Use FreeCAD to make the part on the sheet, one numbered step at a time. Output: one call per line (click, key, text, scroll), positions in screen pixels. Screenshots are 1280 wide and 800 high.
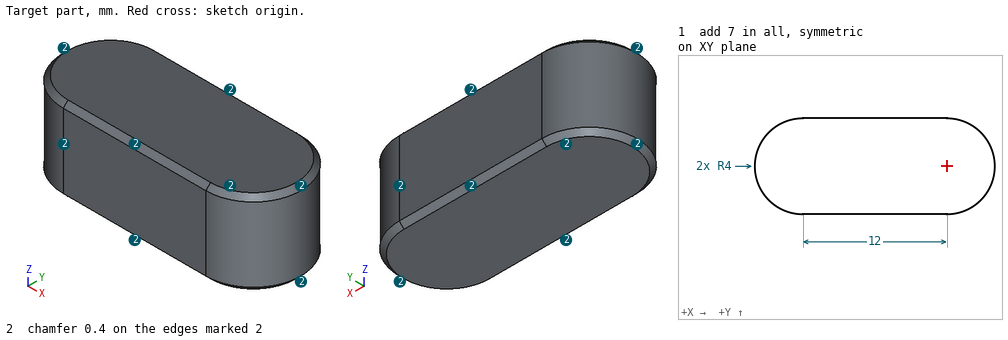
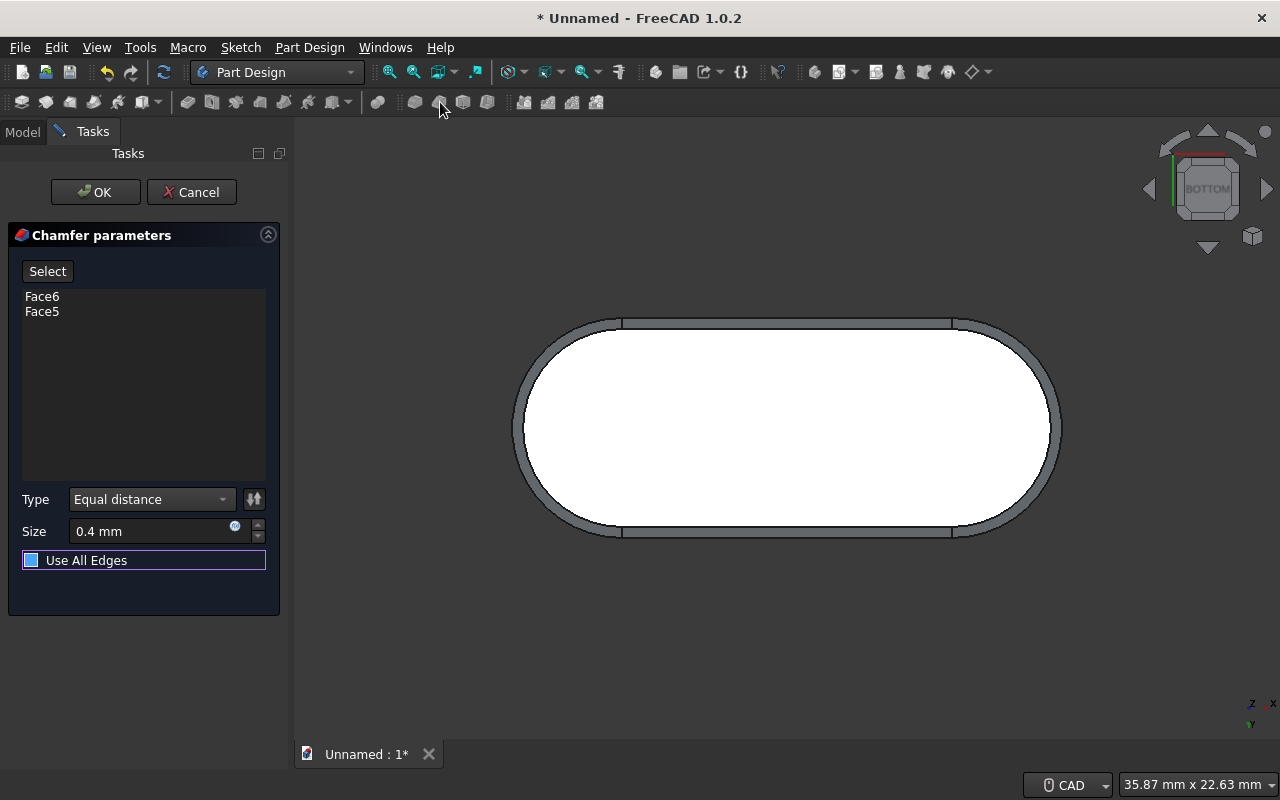
click(96, 192)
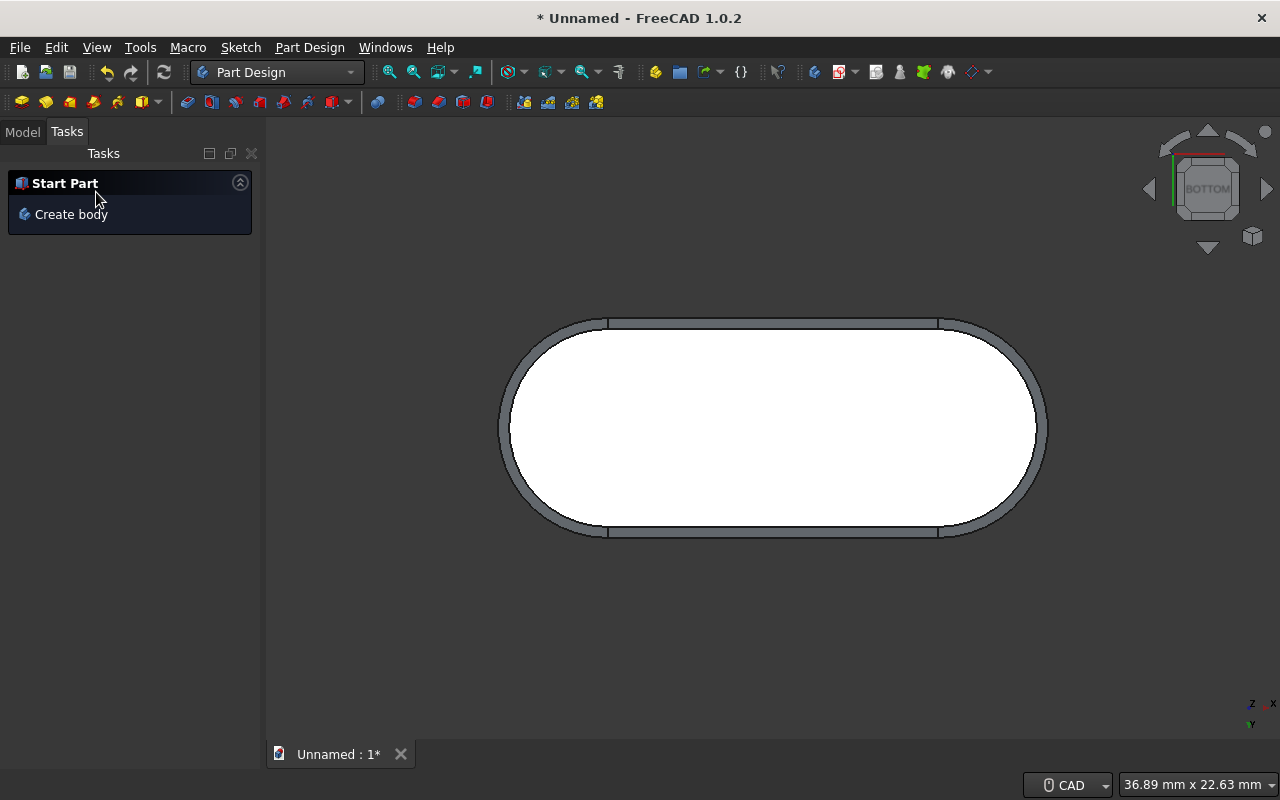
key(0)